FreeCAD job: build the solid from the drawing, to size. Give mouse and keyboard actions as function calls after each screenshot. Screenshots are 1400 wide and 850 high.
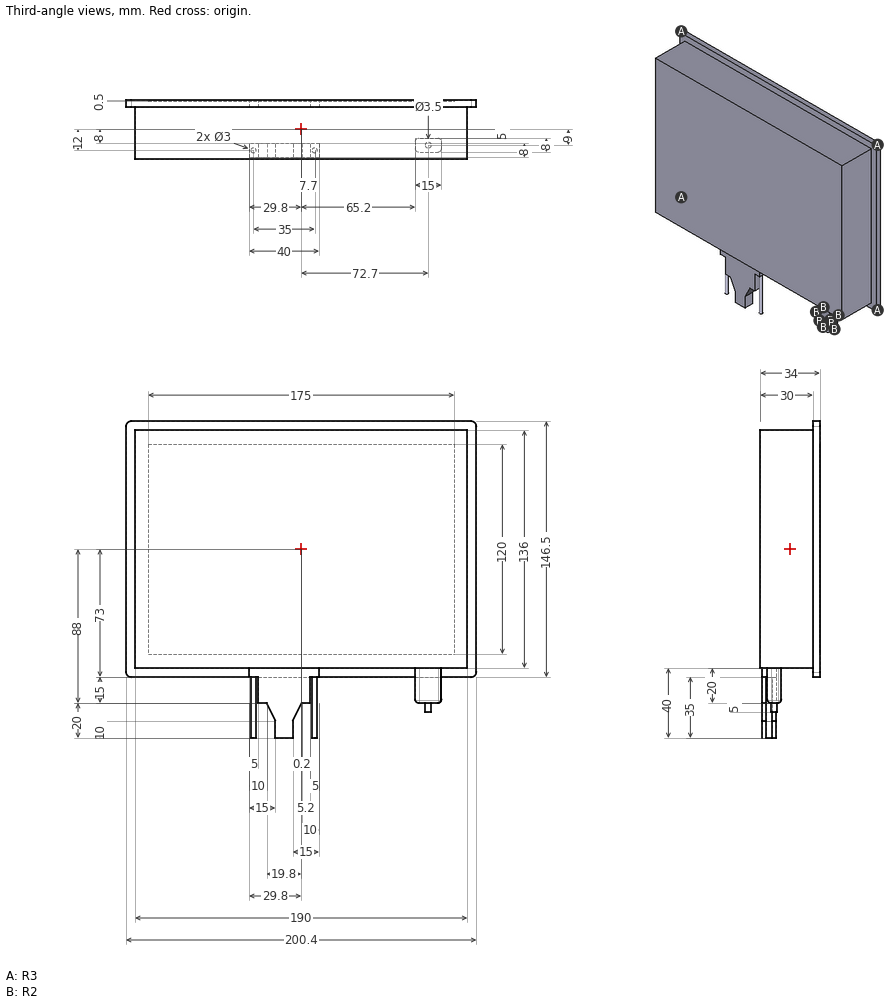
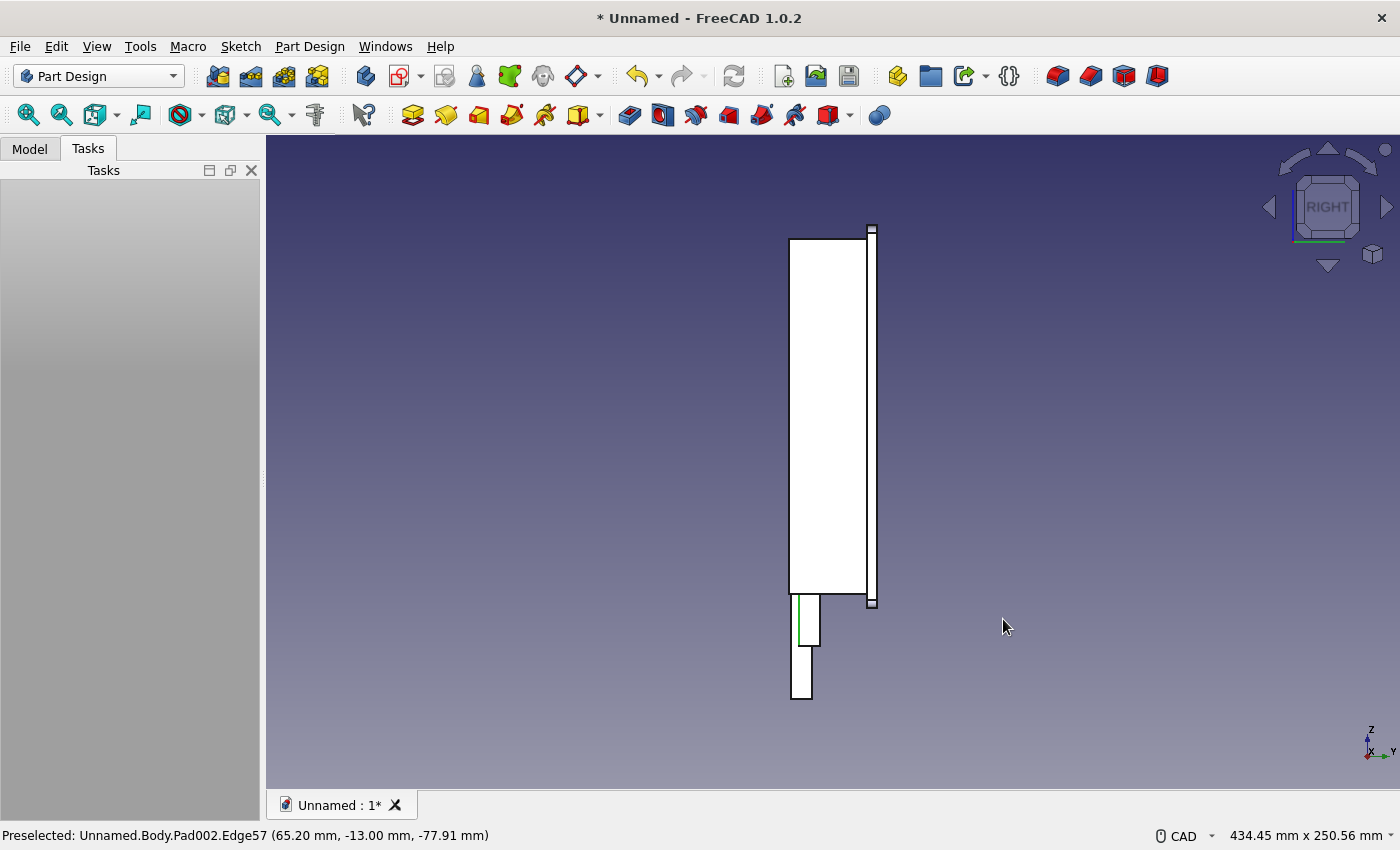
click(820, 619, ctrl)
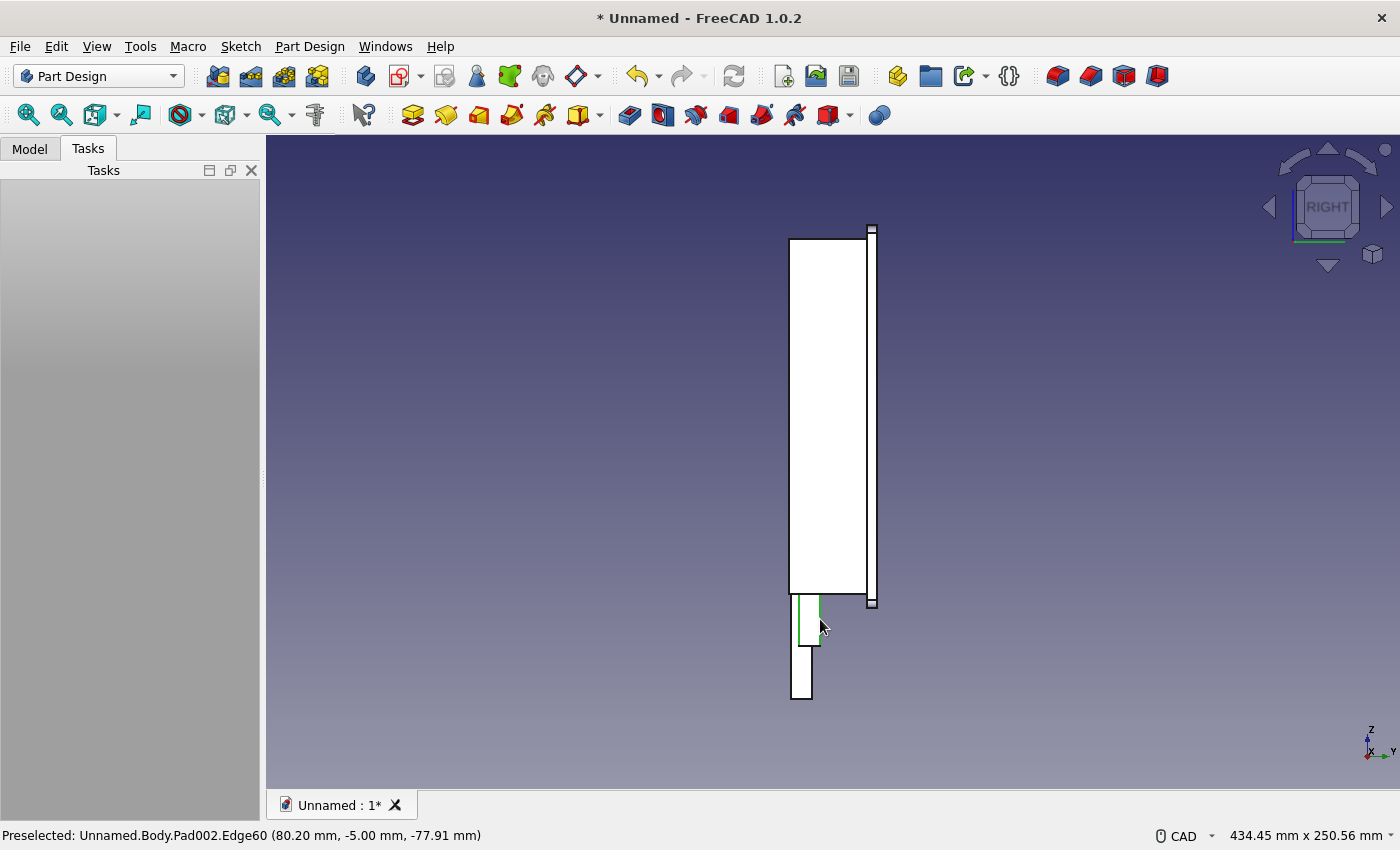
key(5)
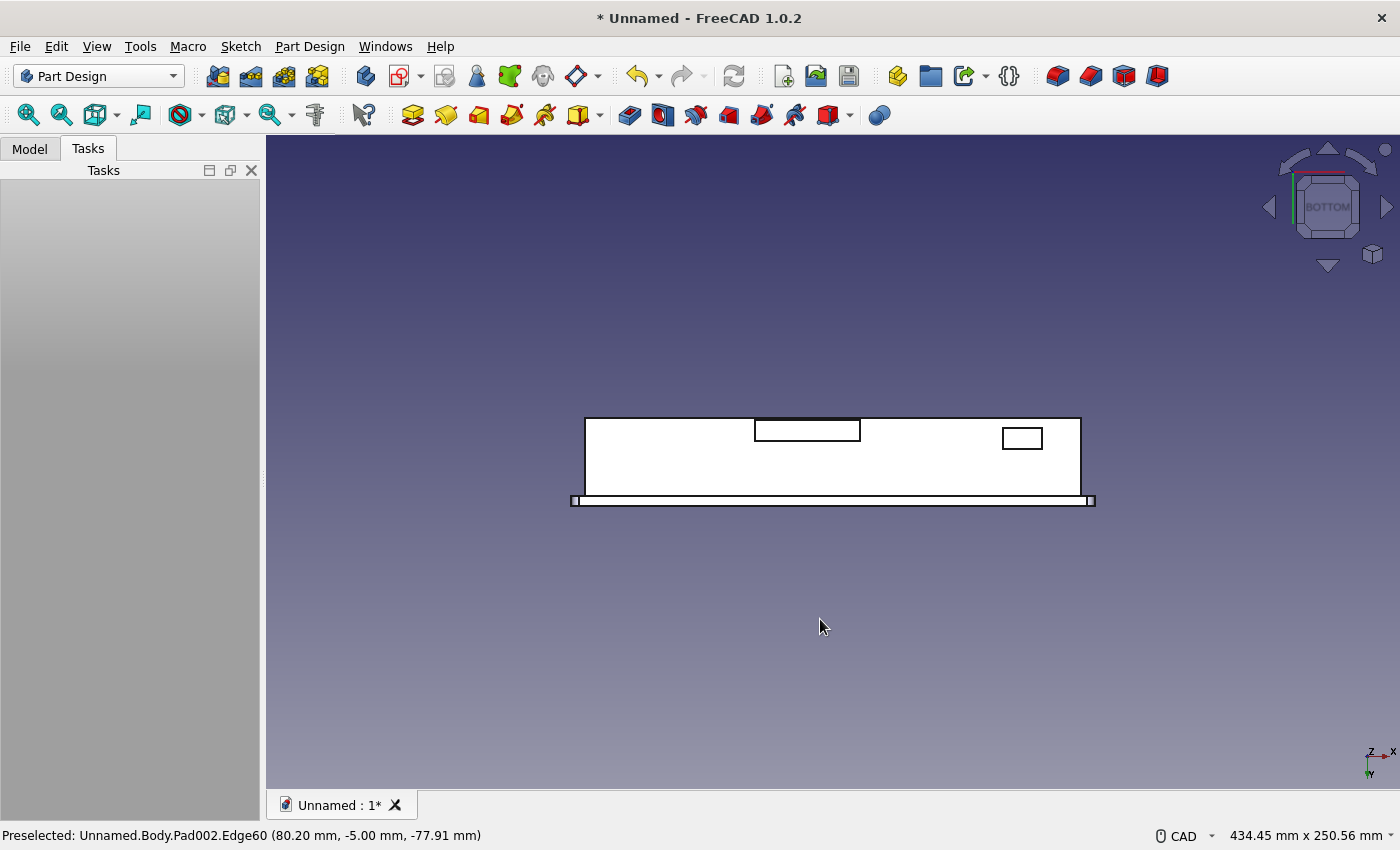
key(4)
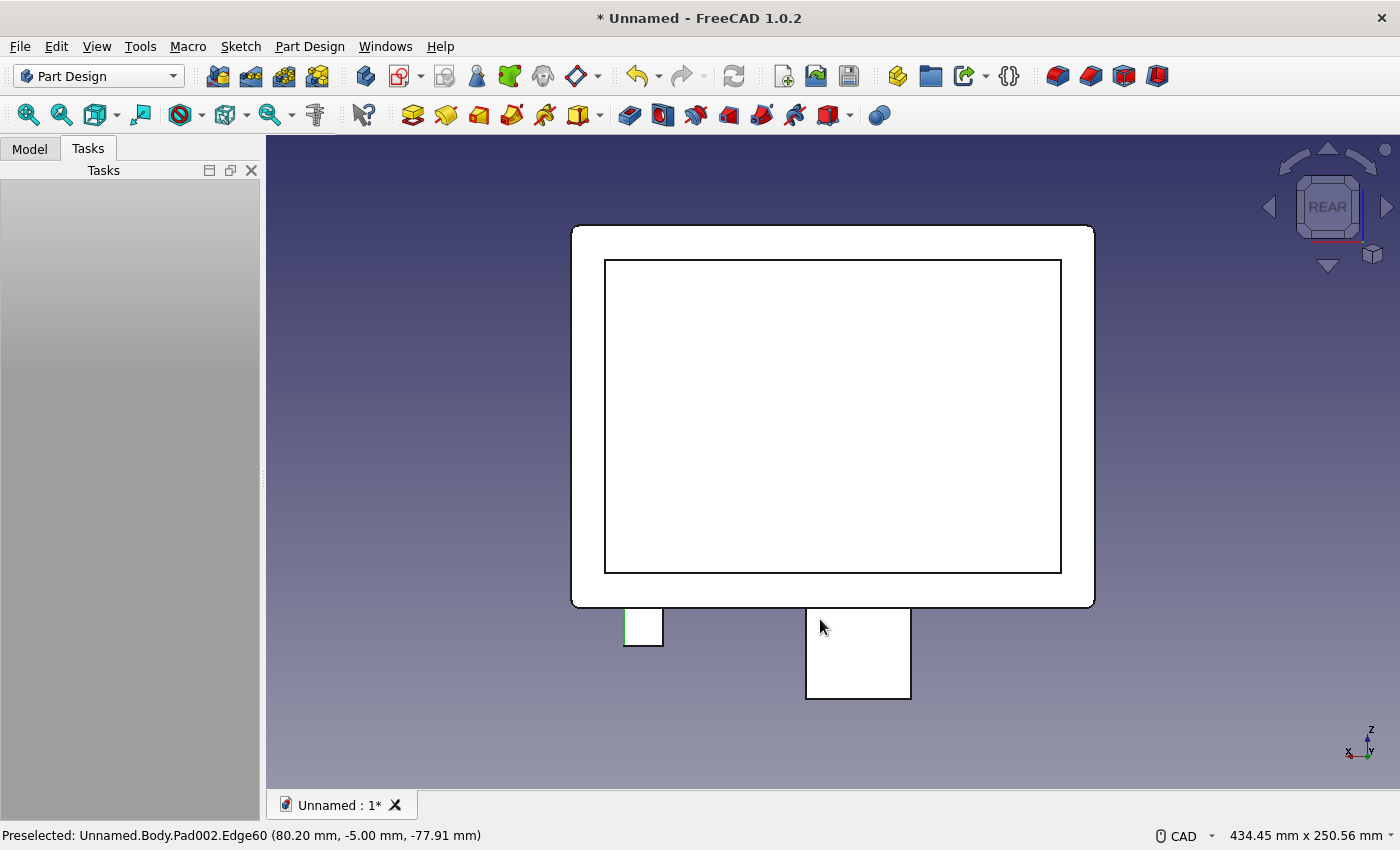
click(663, 619, ctrl)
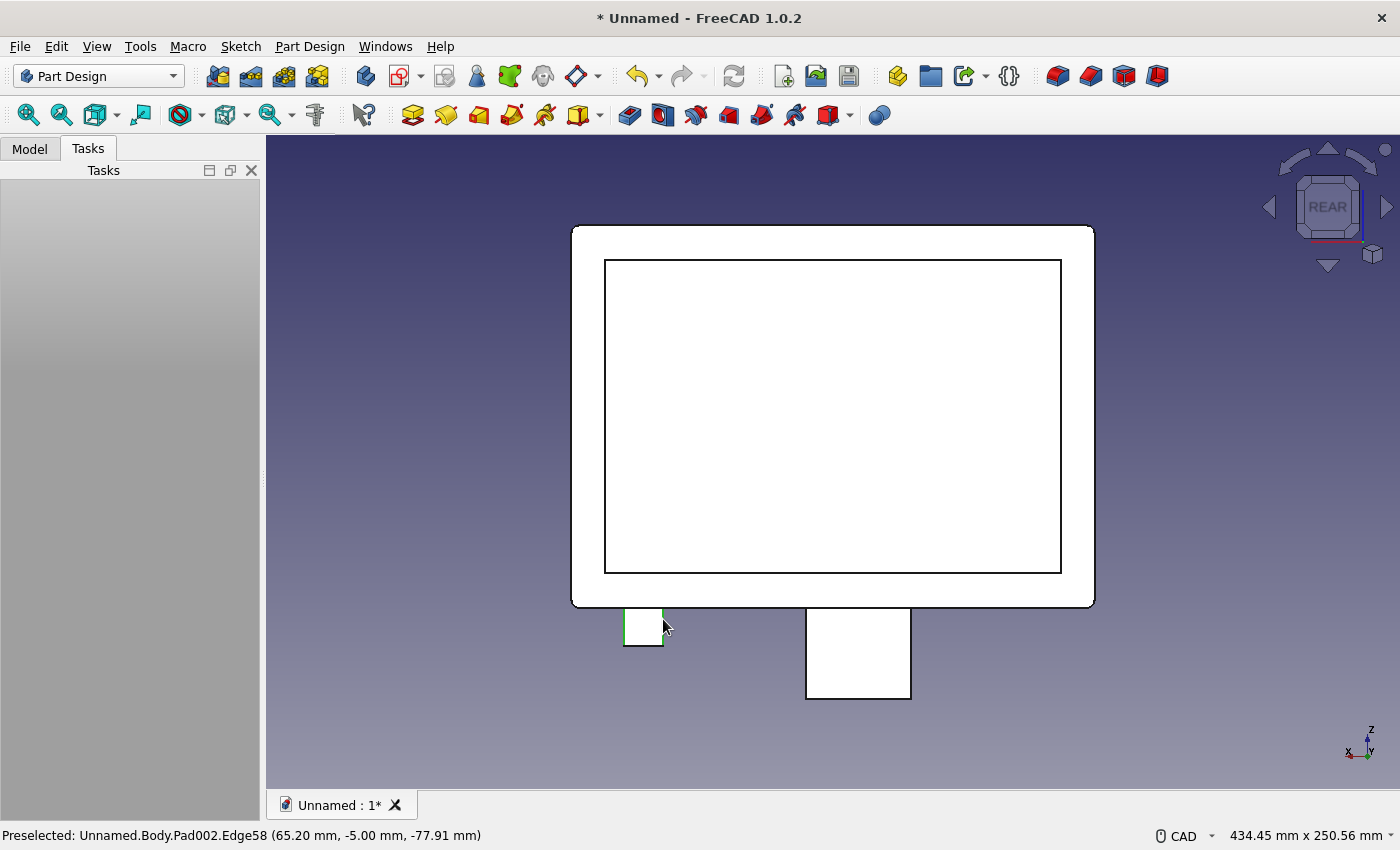
click(1058, 76)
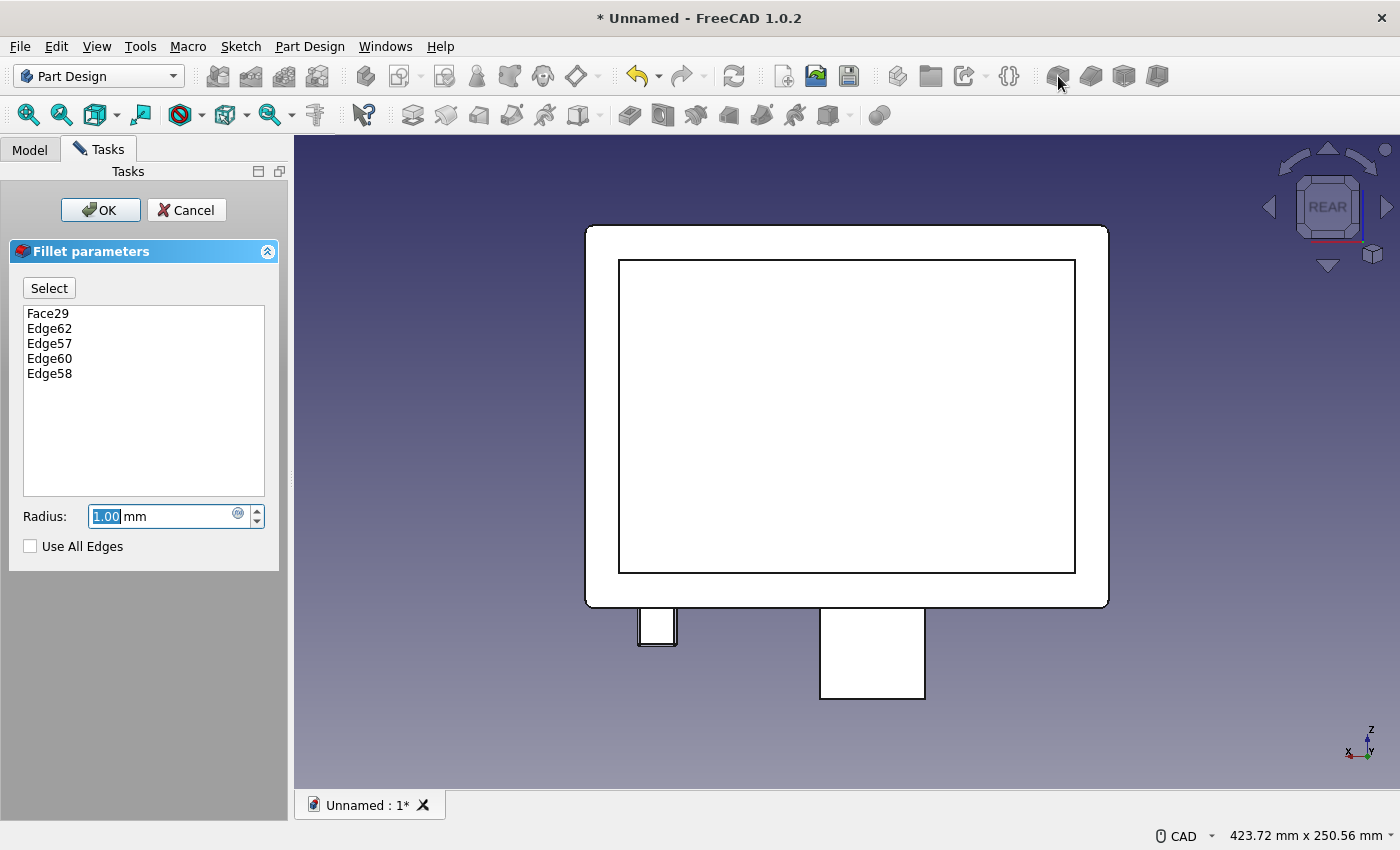
text(2)
key(Tab)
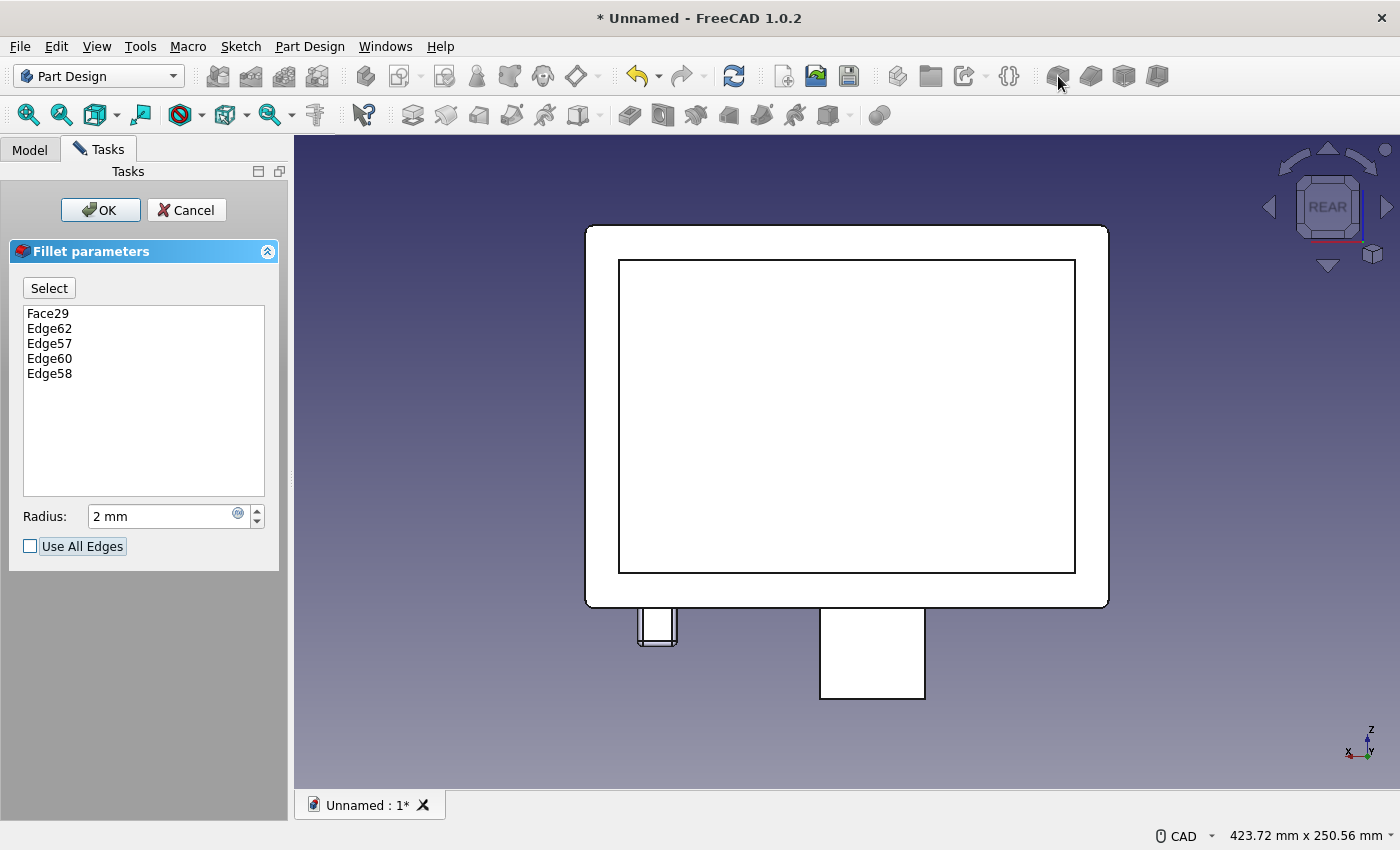
click(101, 210)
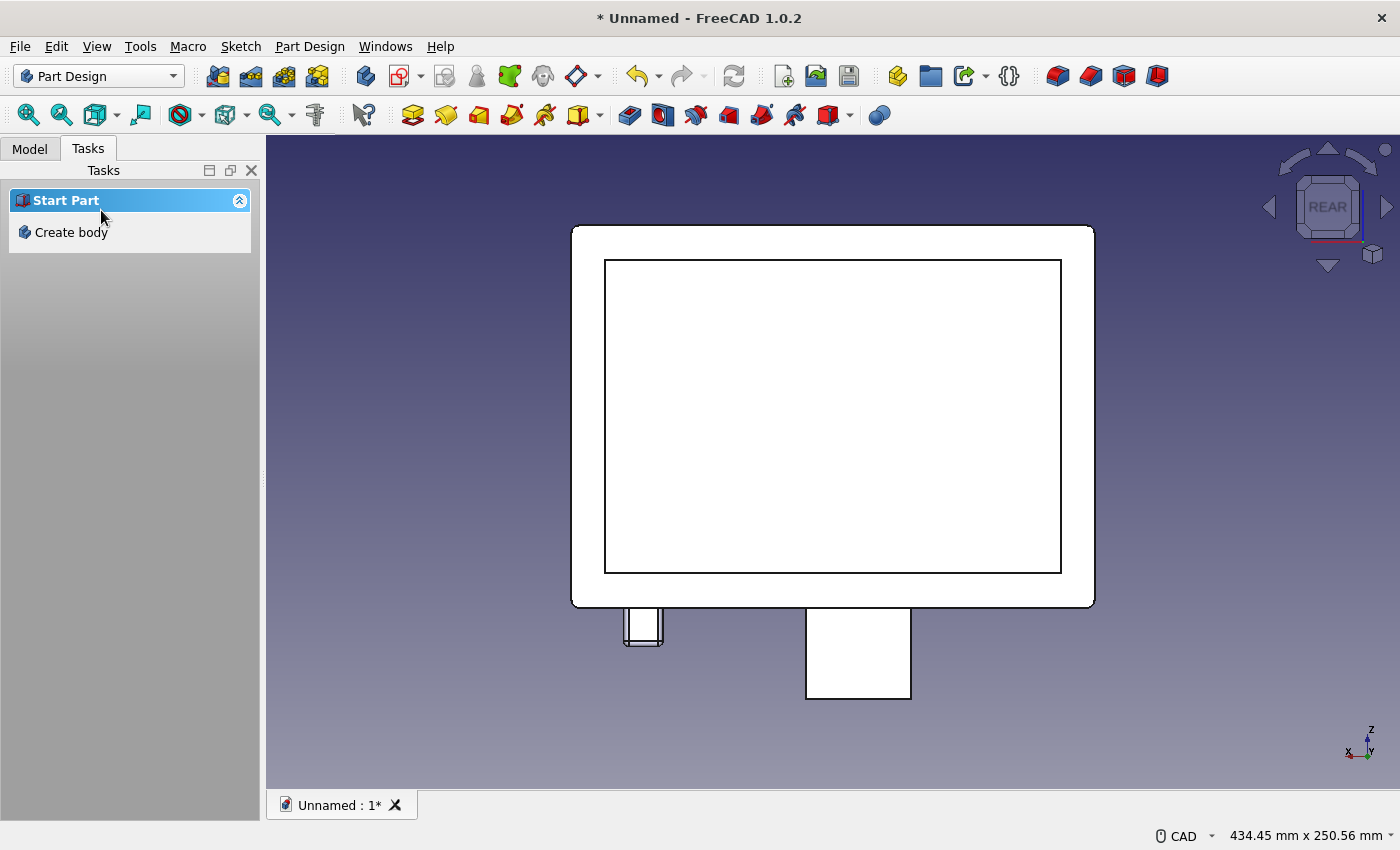
key(5)